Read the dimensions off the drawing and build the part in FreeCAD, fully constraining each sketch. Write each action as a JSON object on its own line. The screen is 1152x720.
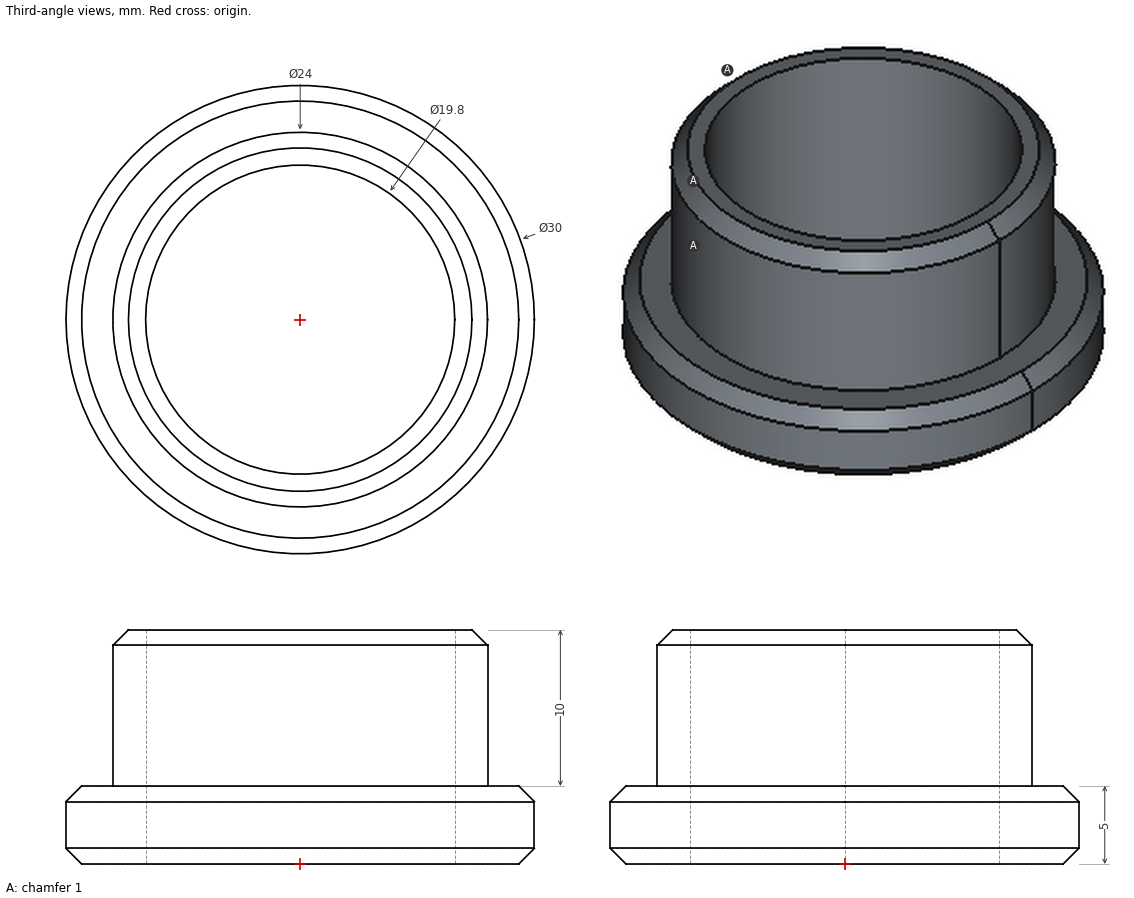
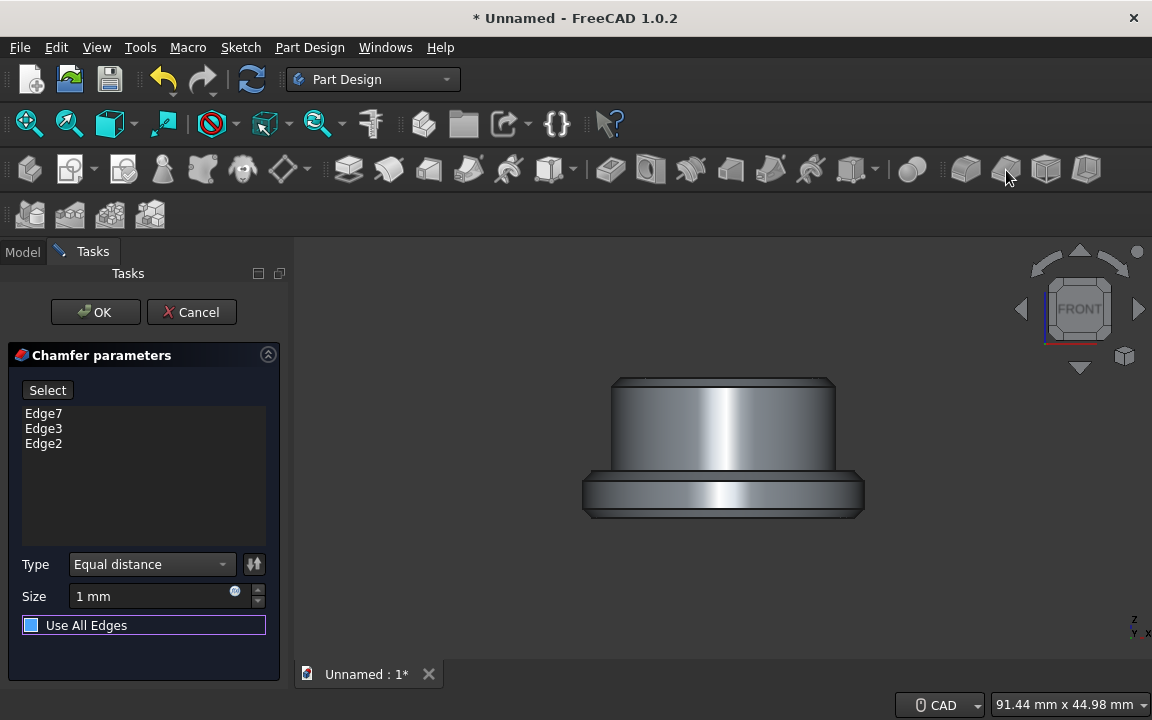
{"action": "left_click", "coordinate": [96, 312]}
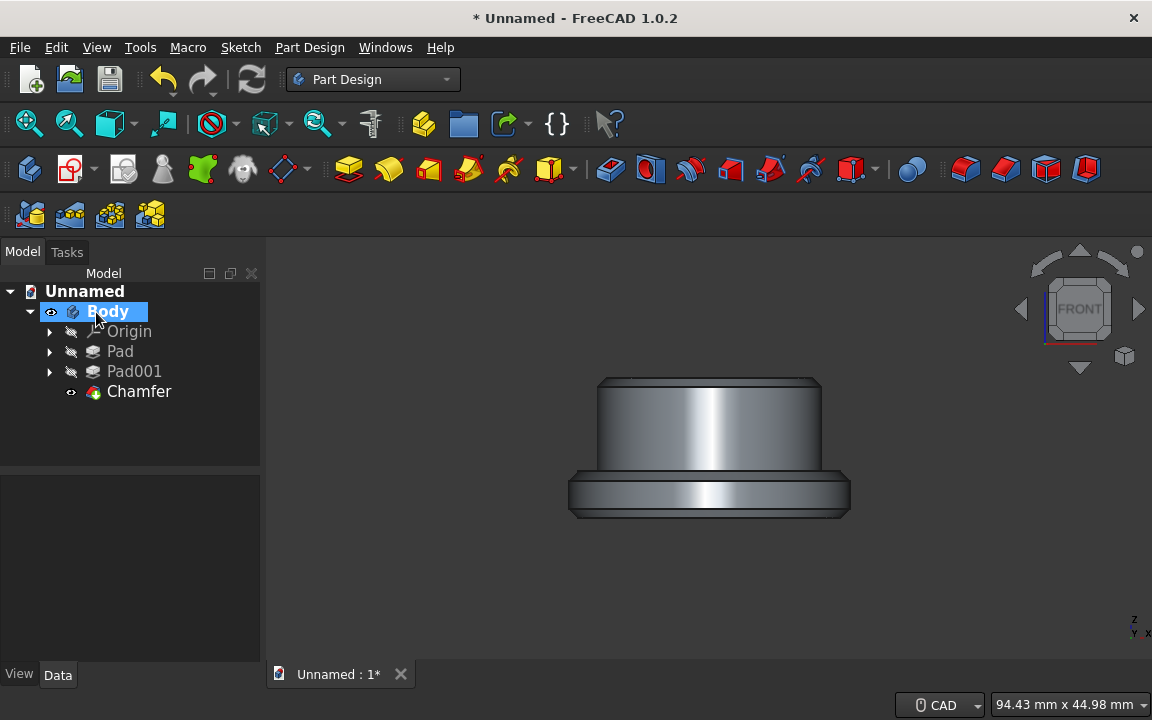
{"action": "key", "text": "0"}